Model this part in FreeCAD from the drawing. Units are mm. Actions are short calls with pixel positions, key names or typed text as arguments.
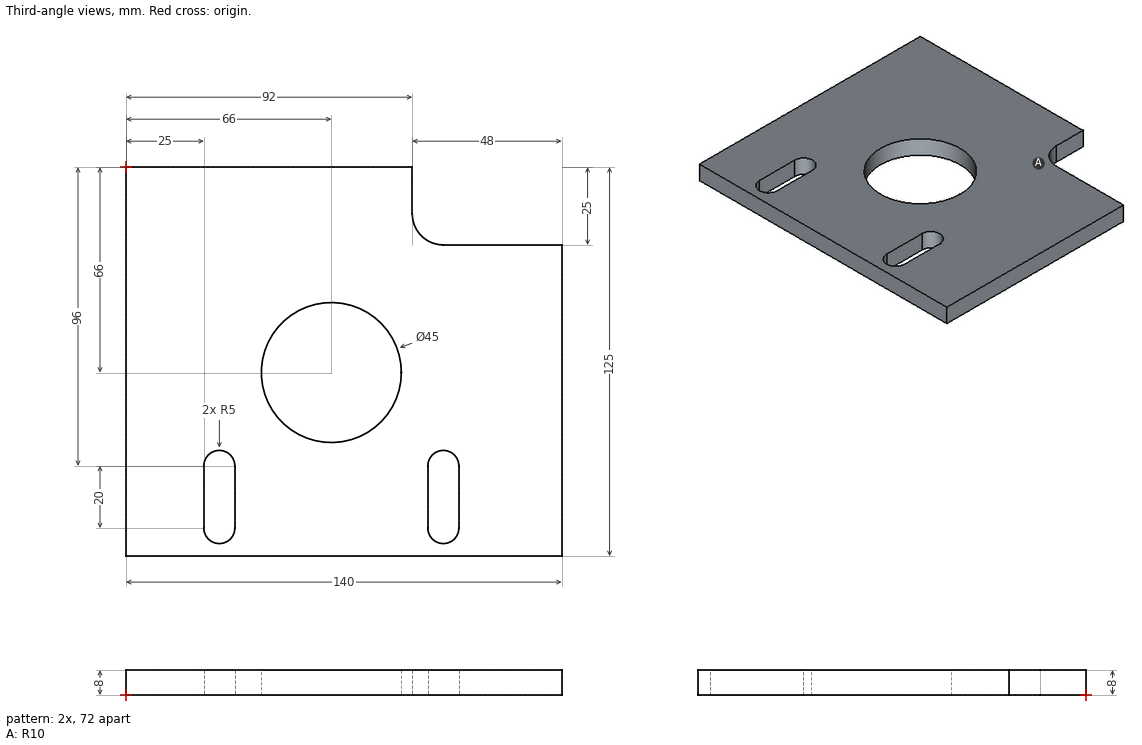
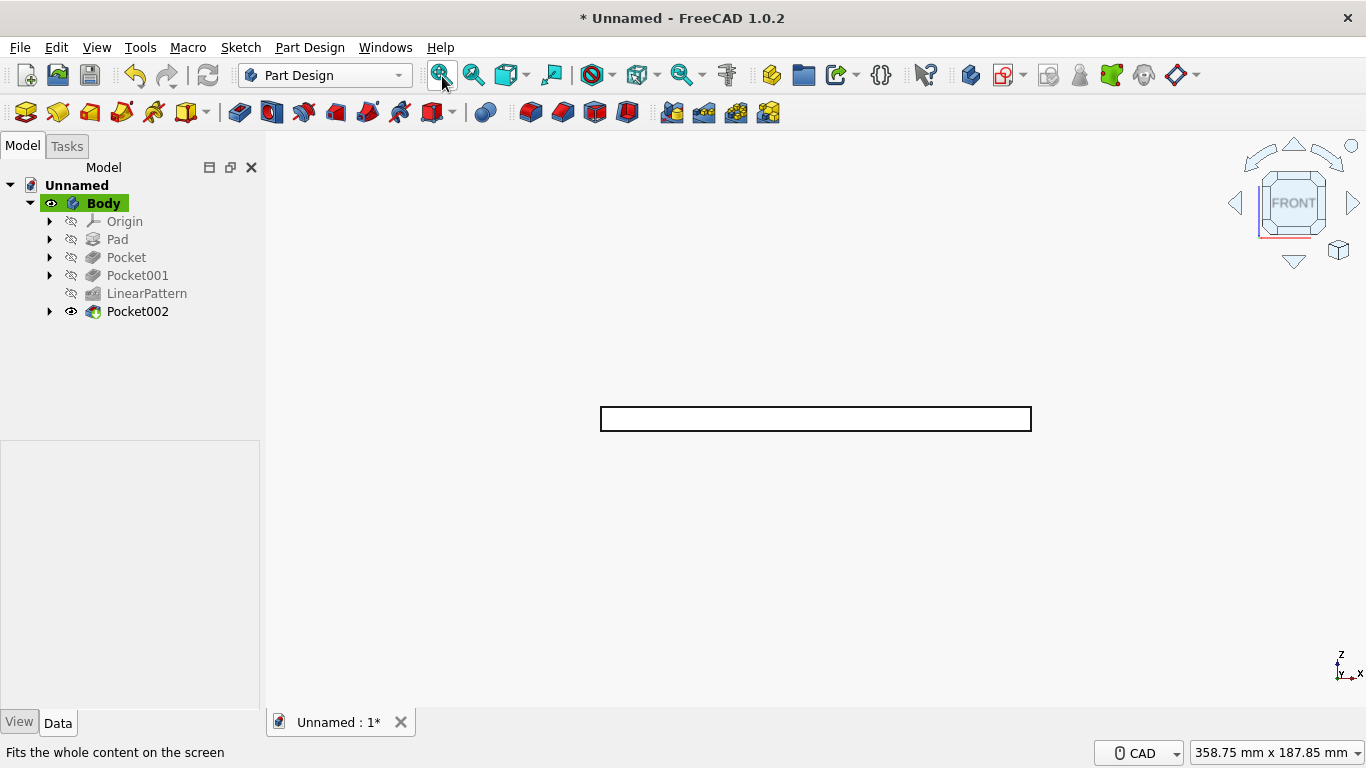
key(3)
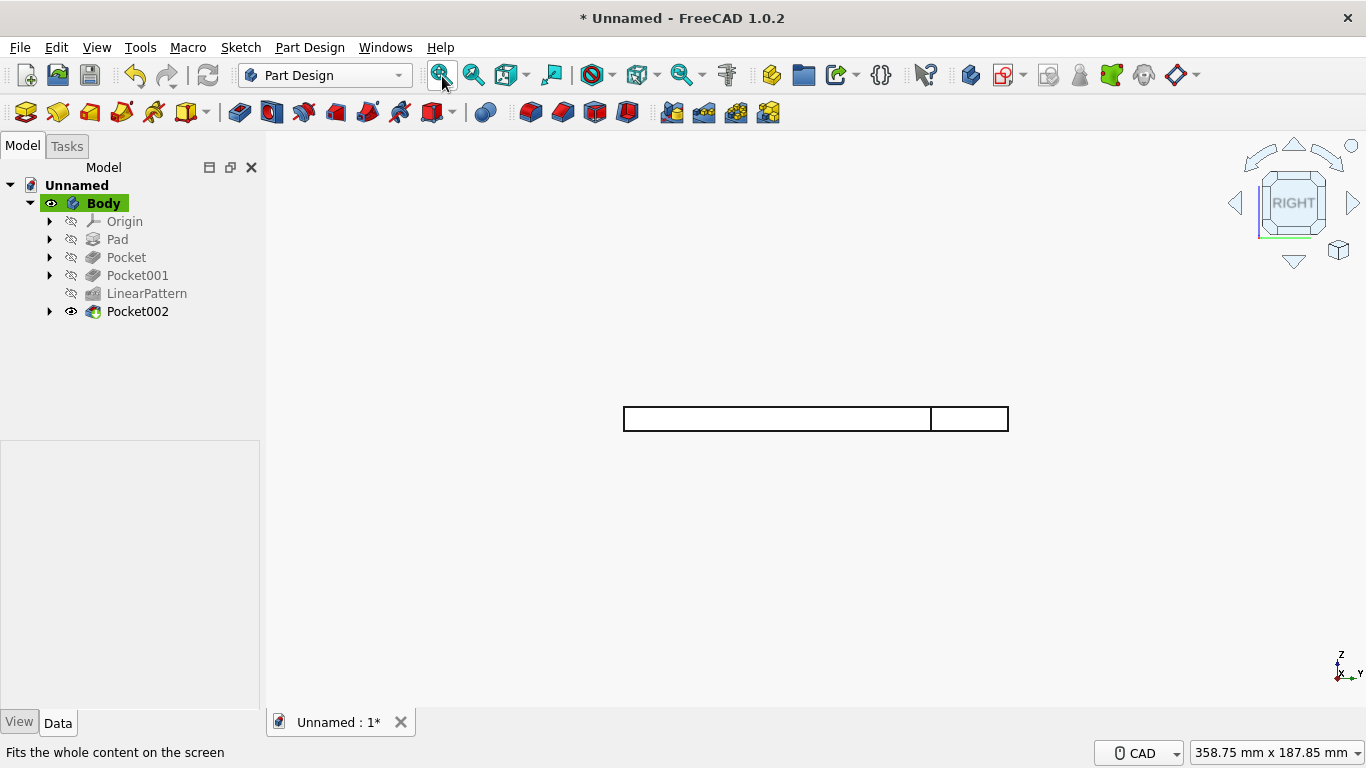
key(v)
key(f)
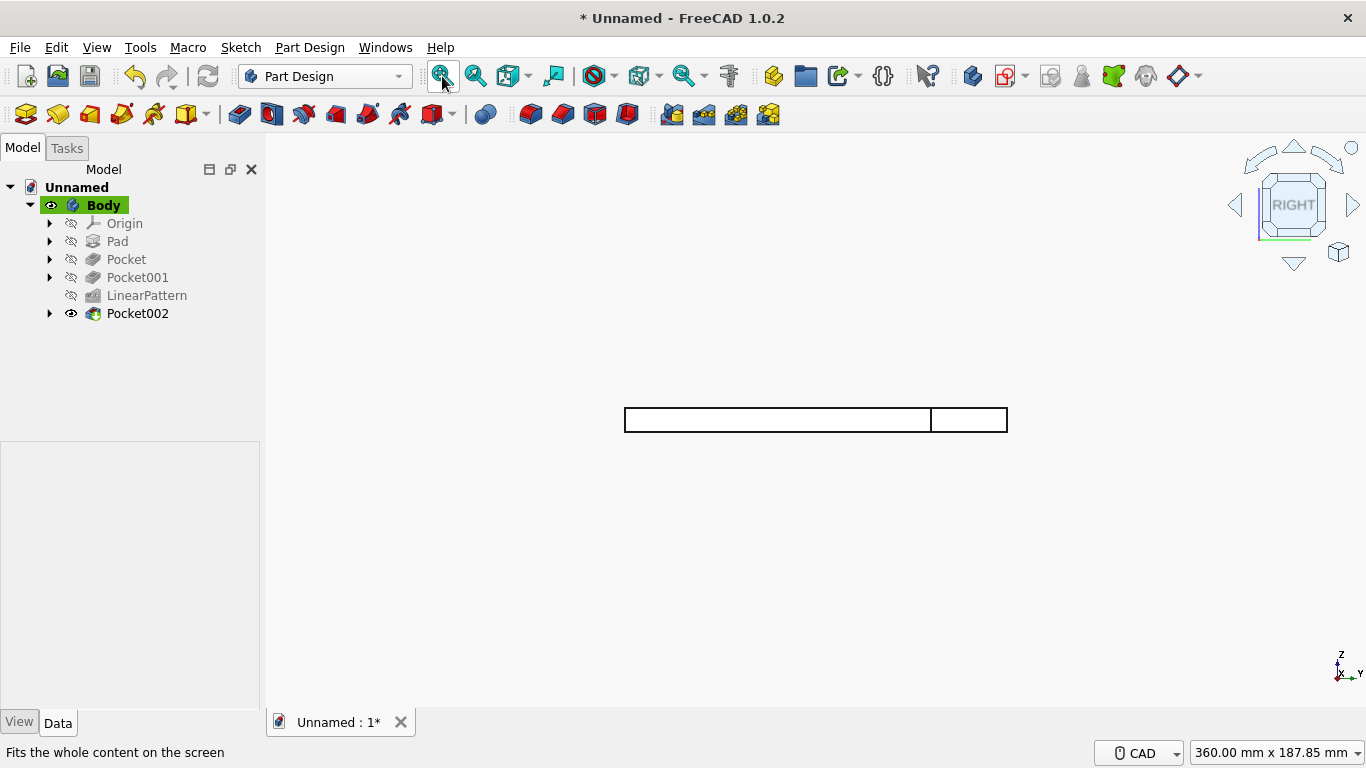
key(5)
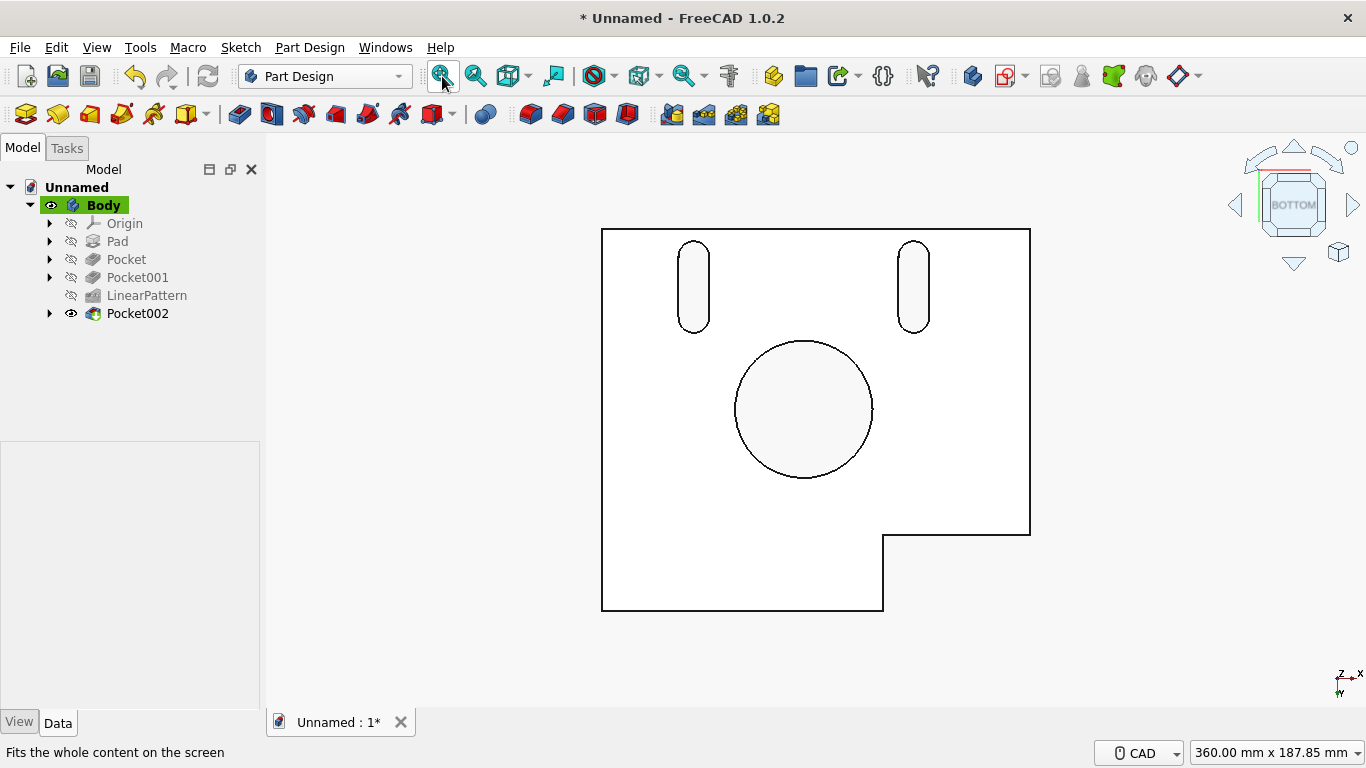
key(4)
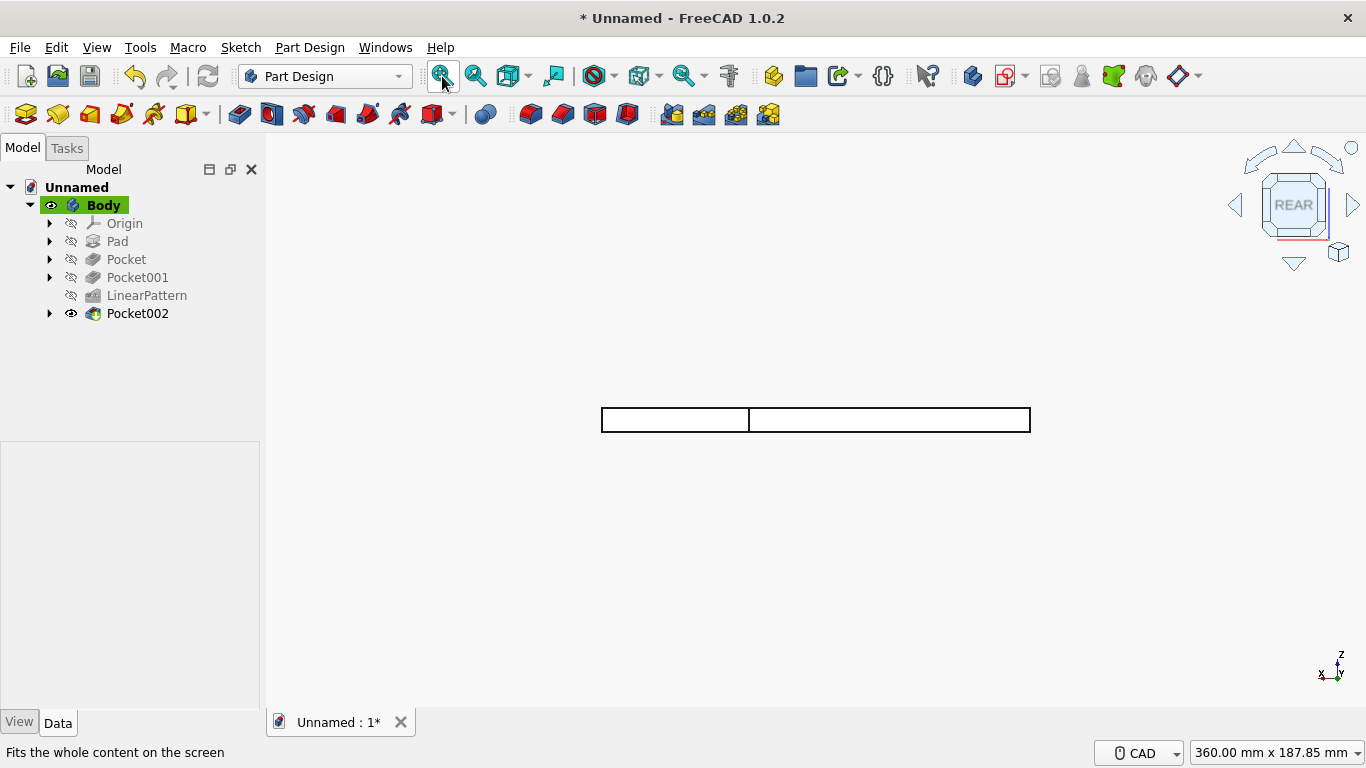
key(v)
key(f)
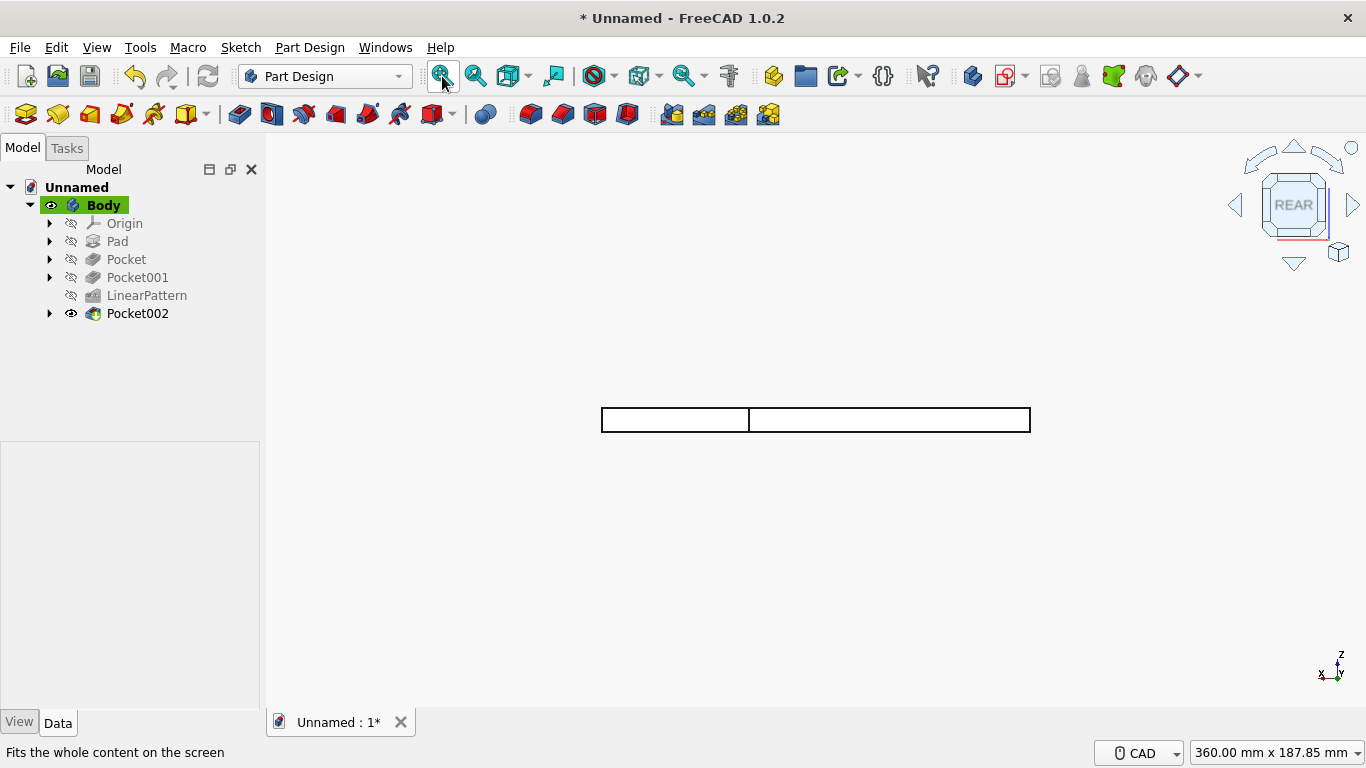
key(6)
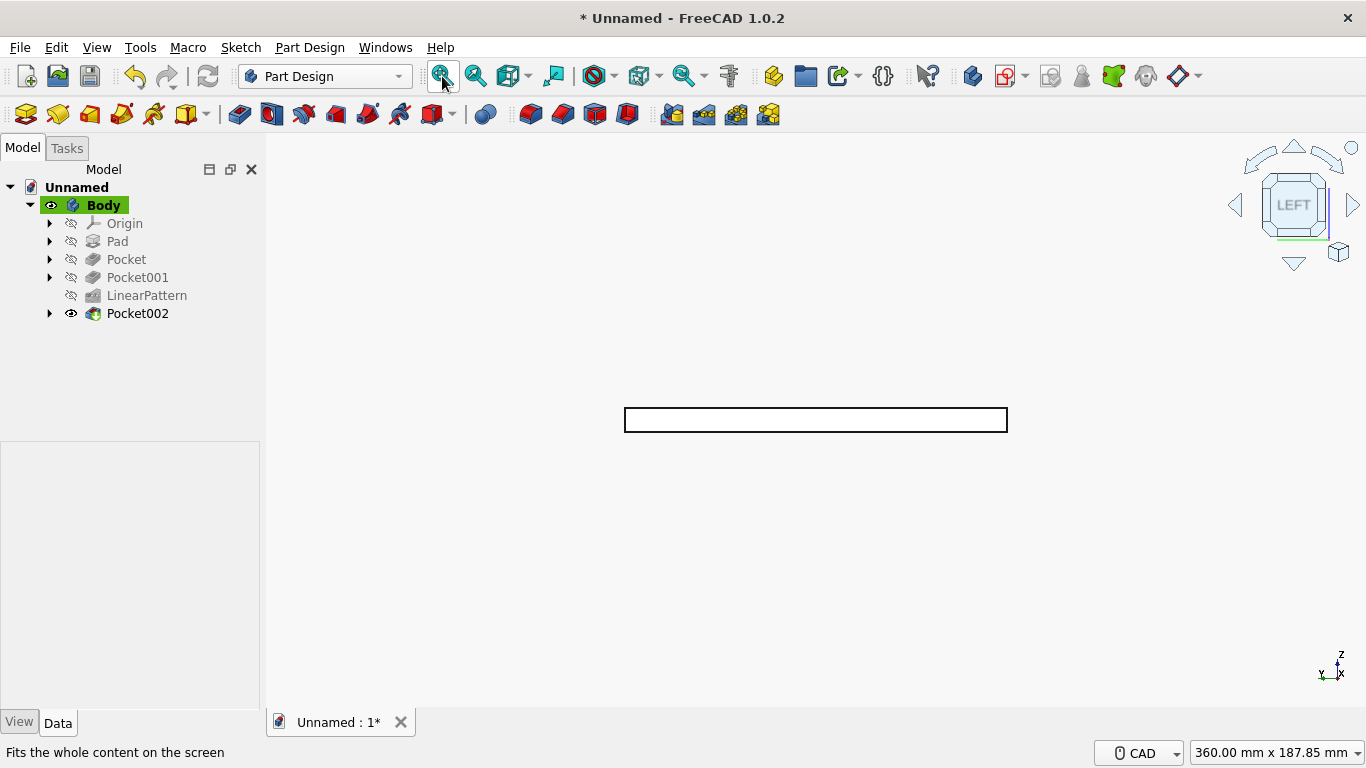
click(444, 76)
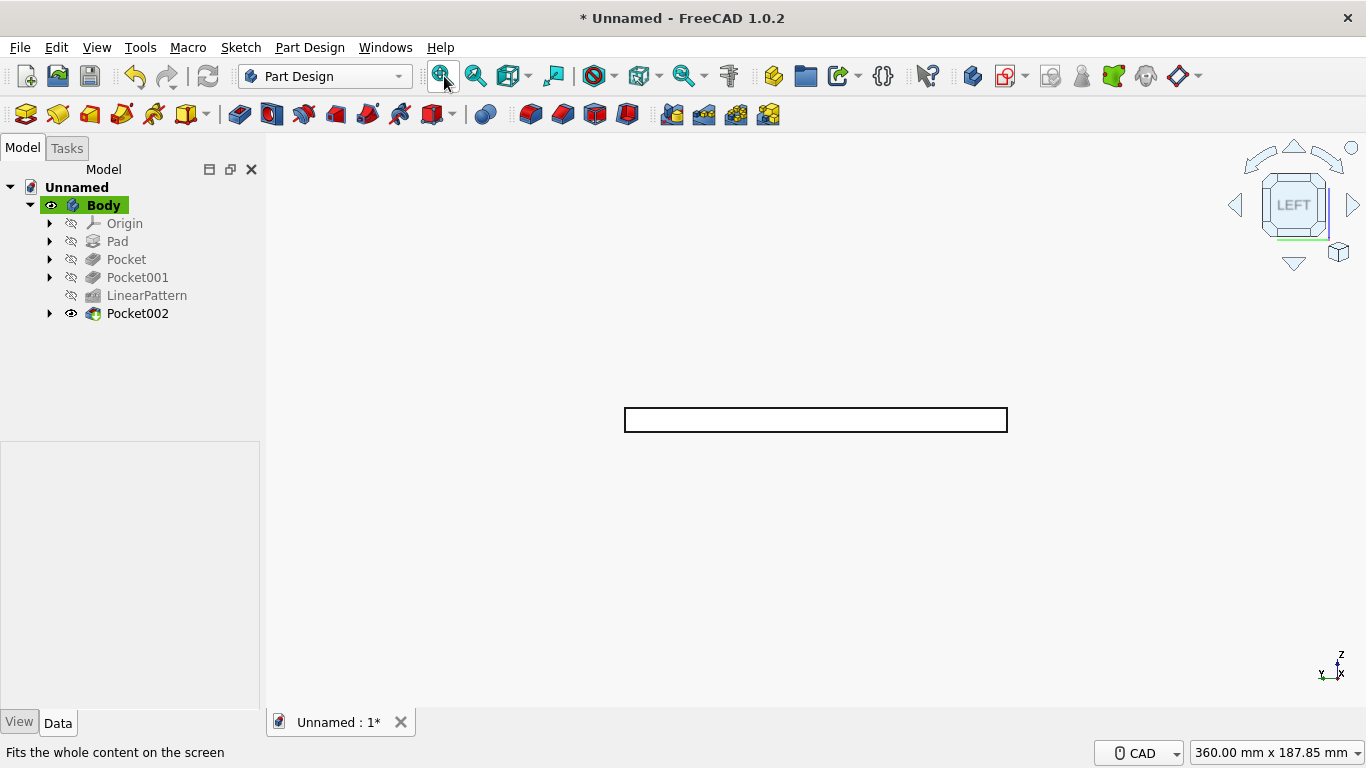
key(v)
key(3)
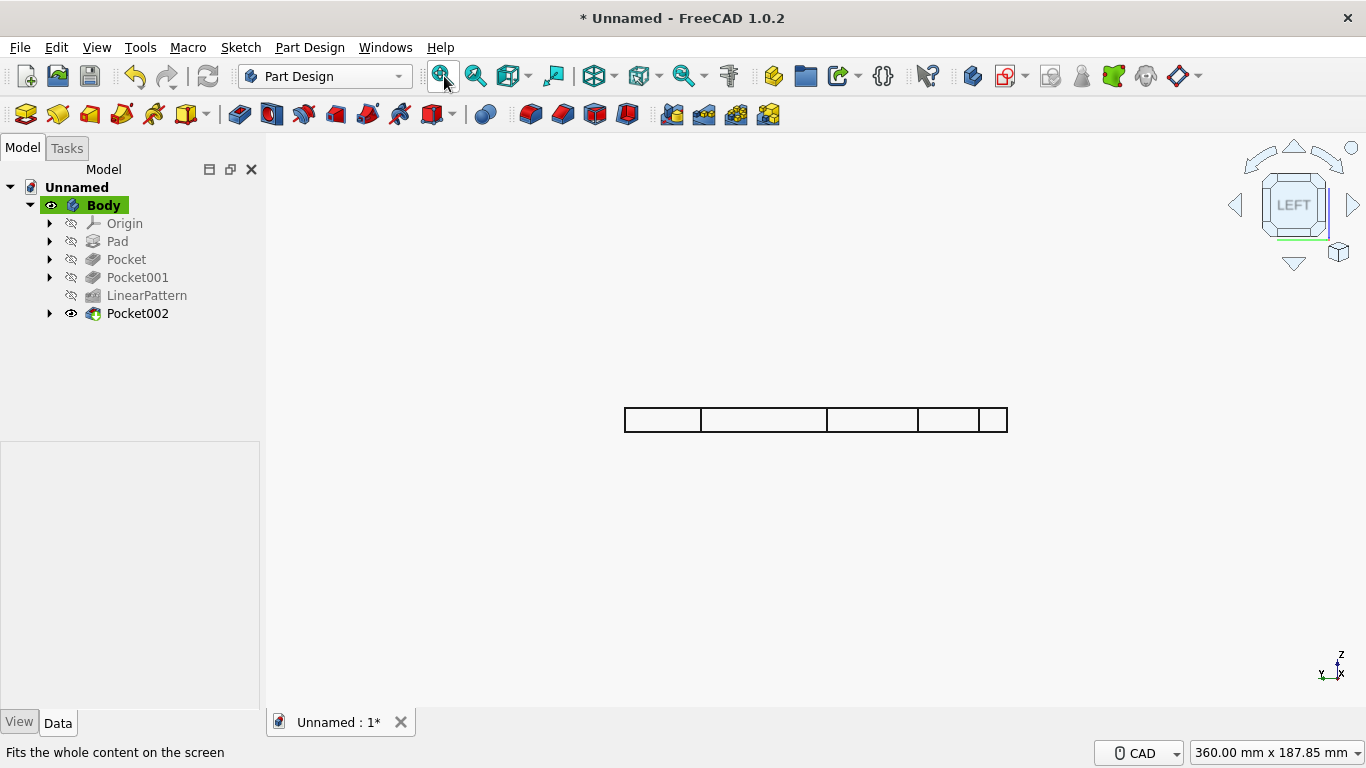
key(0)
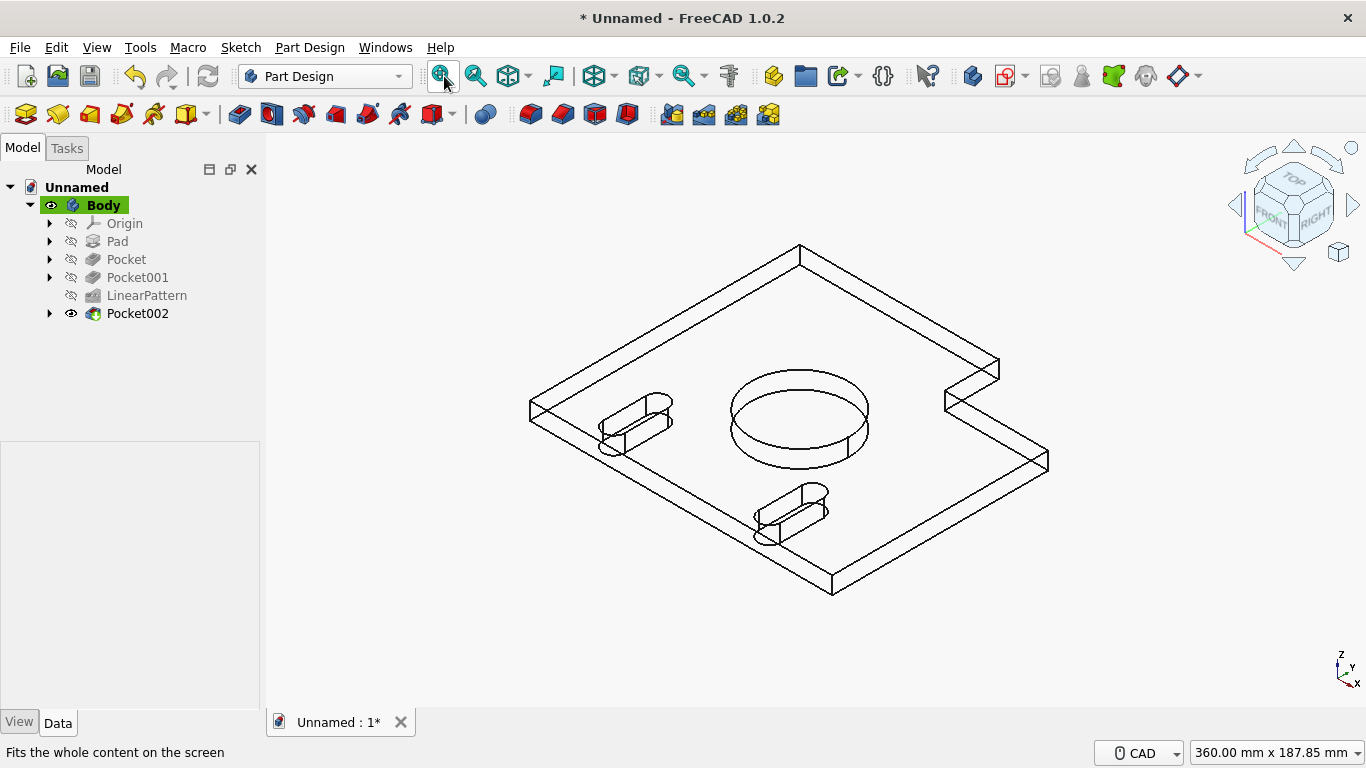
click(945, 400)